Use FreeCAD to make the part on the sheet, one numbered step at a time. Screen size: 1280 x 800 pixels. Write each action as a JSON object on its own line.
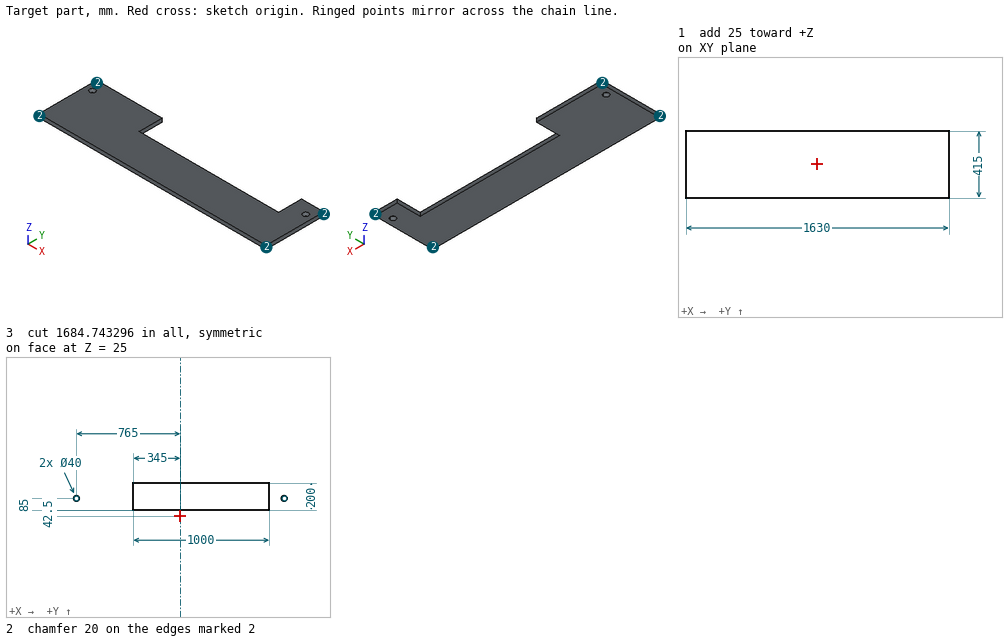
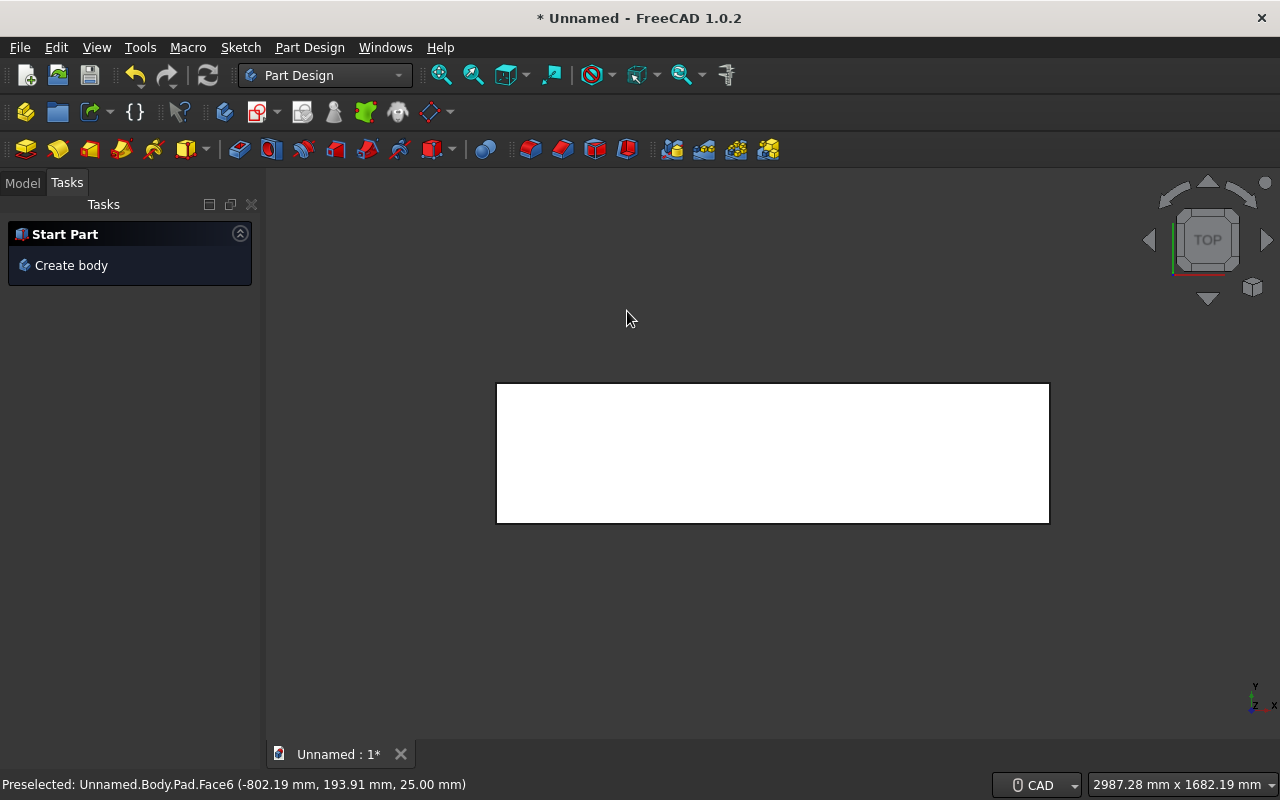
{"action": "scroll", "coordinate": [496, 382], "scroll_direction": "up", "scroll_amount": 8}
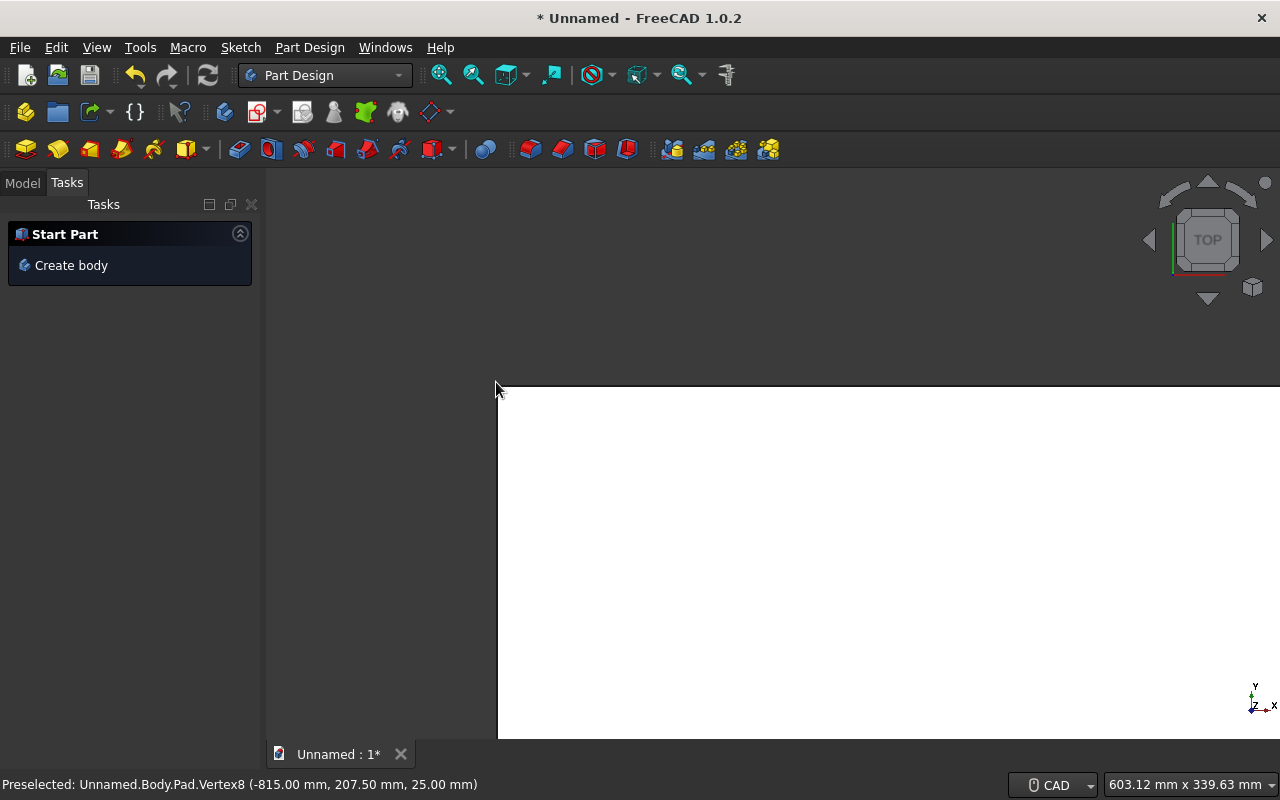
{"action": "left_click", "coordinate": [442, 76]}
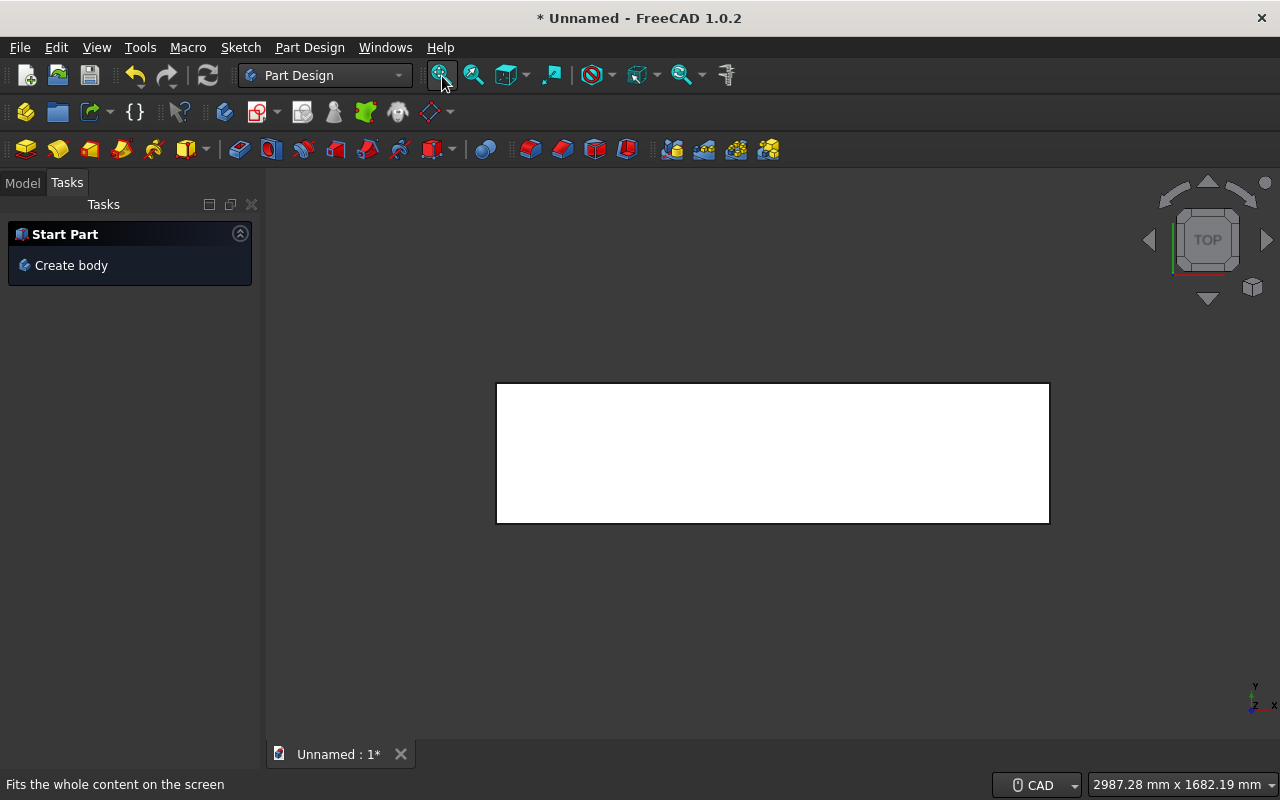
{"action": "key", "text": "1"}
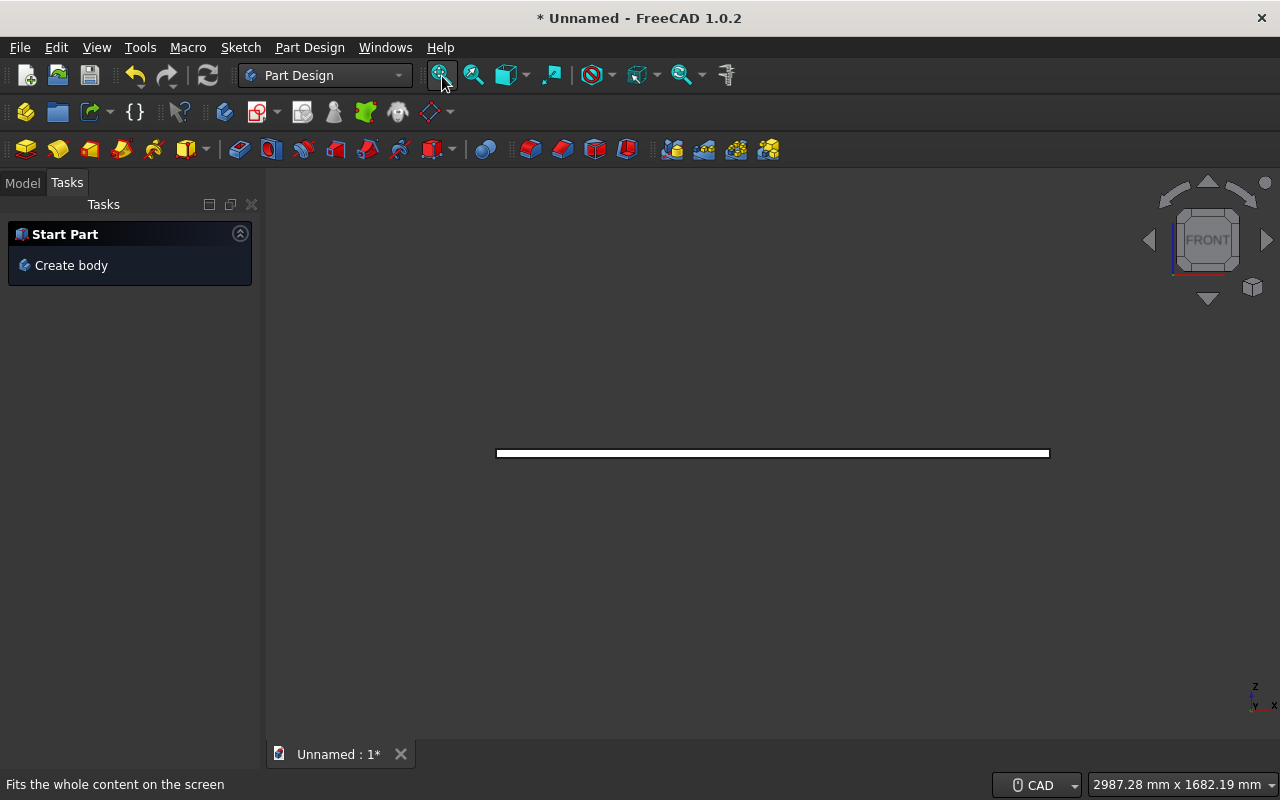
{"action": "scroll", "coordinate": [496, 453], "scroll_direction": "up", "scroll_amount": 8}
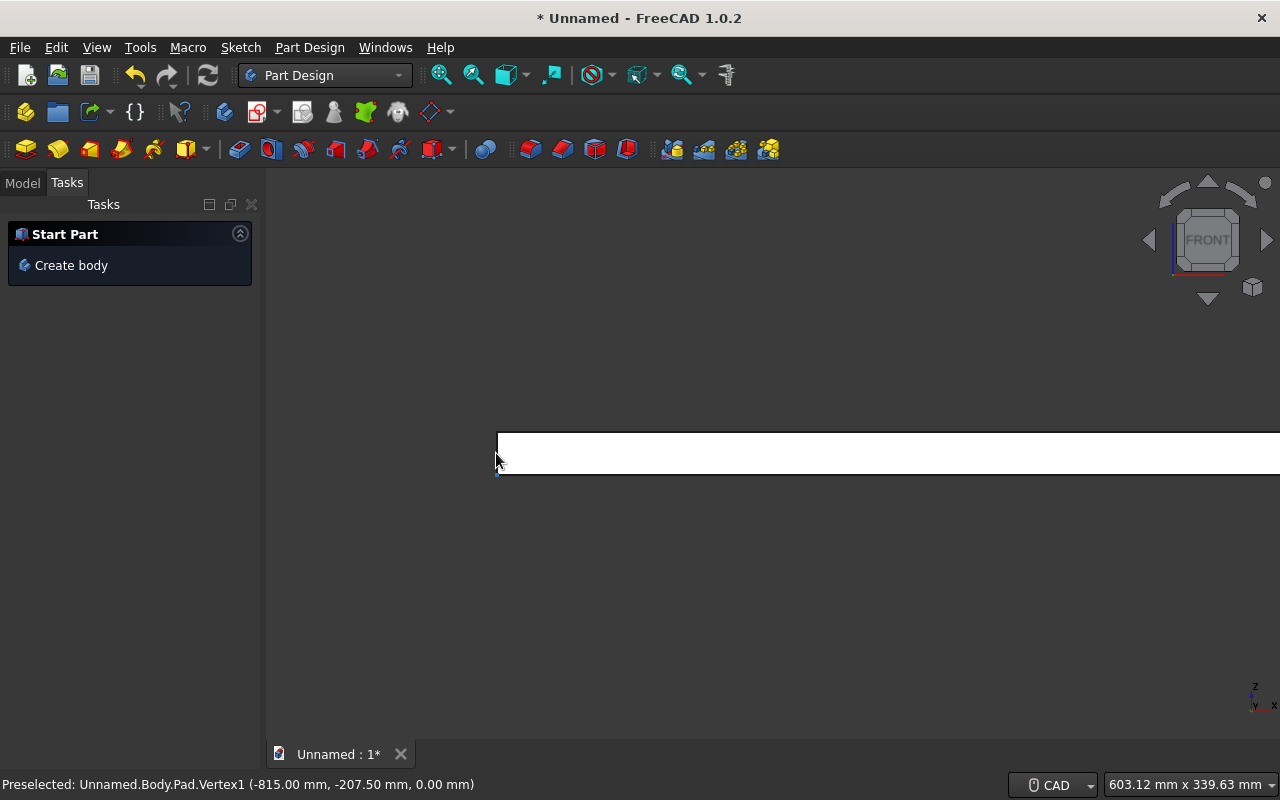
{"action": "left_click", "coordinate": [497, 453]}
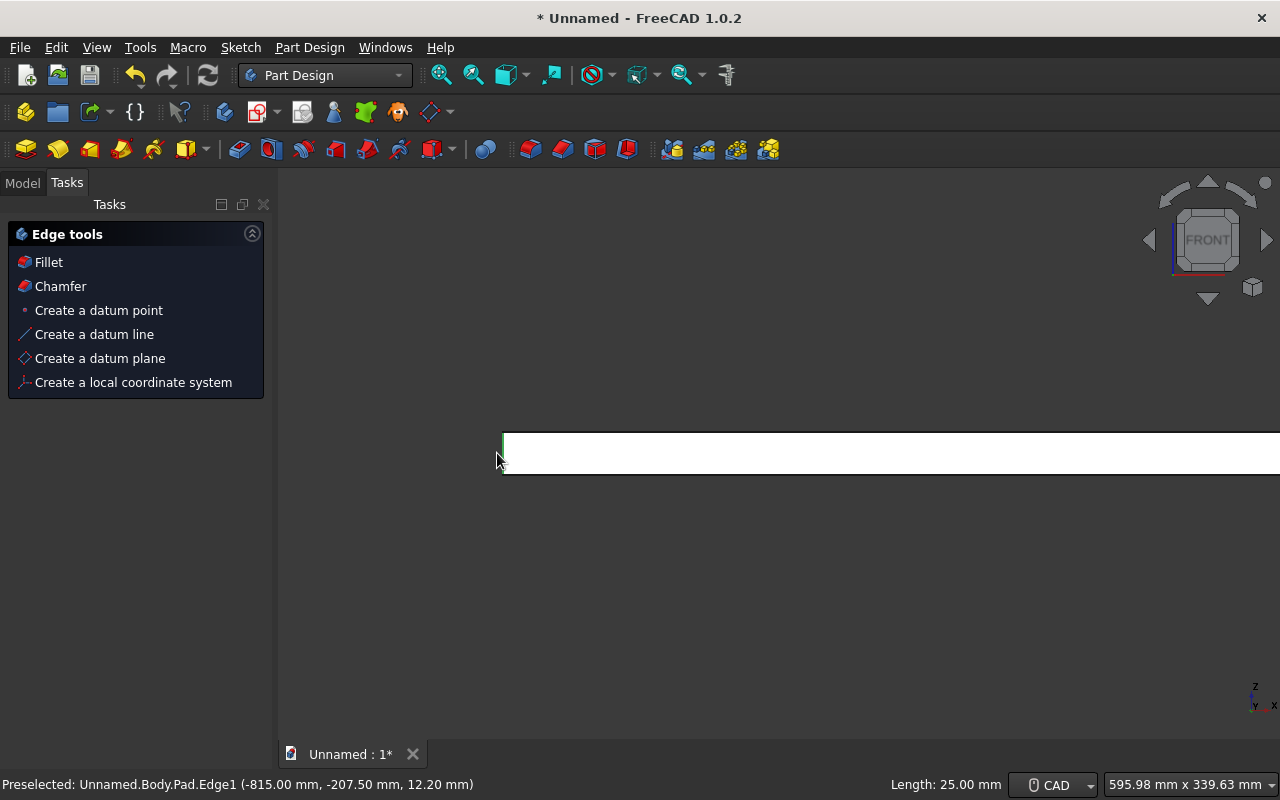
{"action": "left_click", "coordinate": [442, 76]}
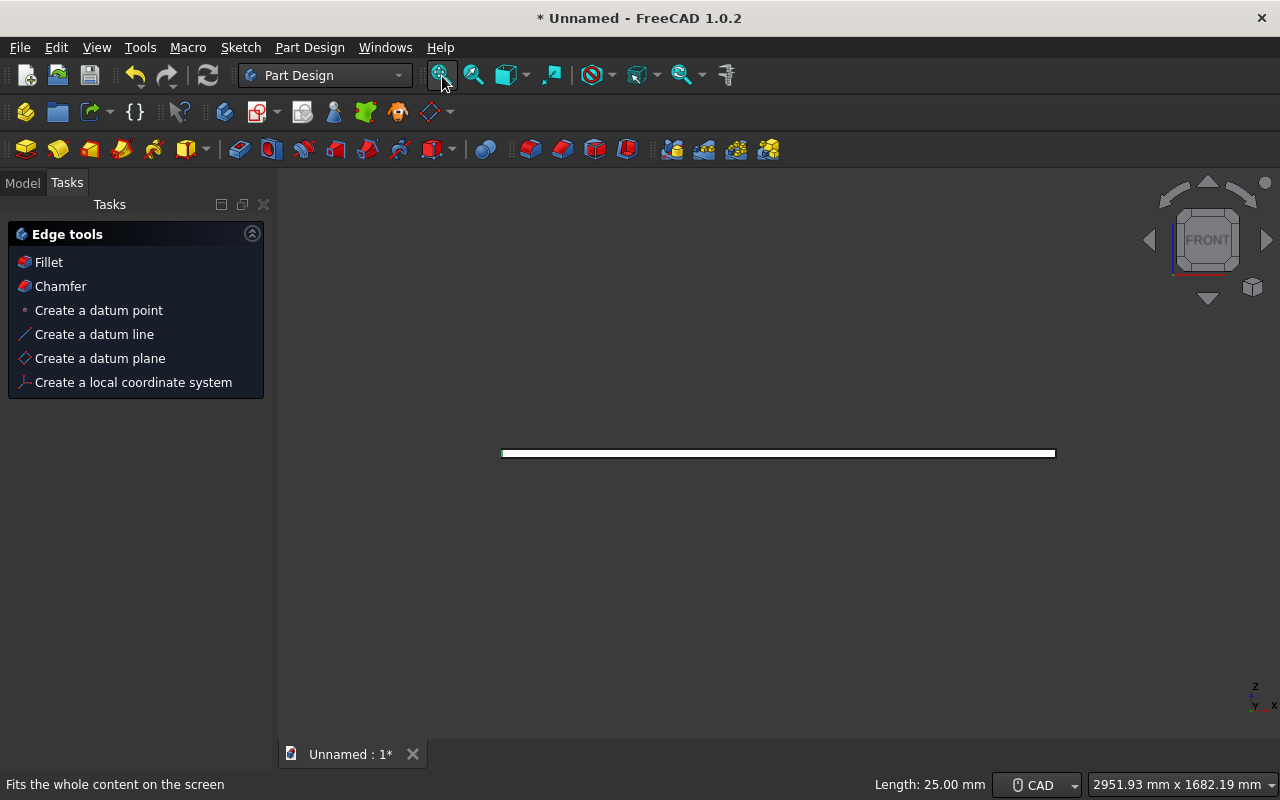
{"action": "key", "text": "3"}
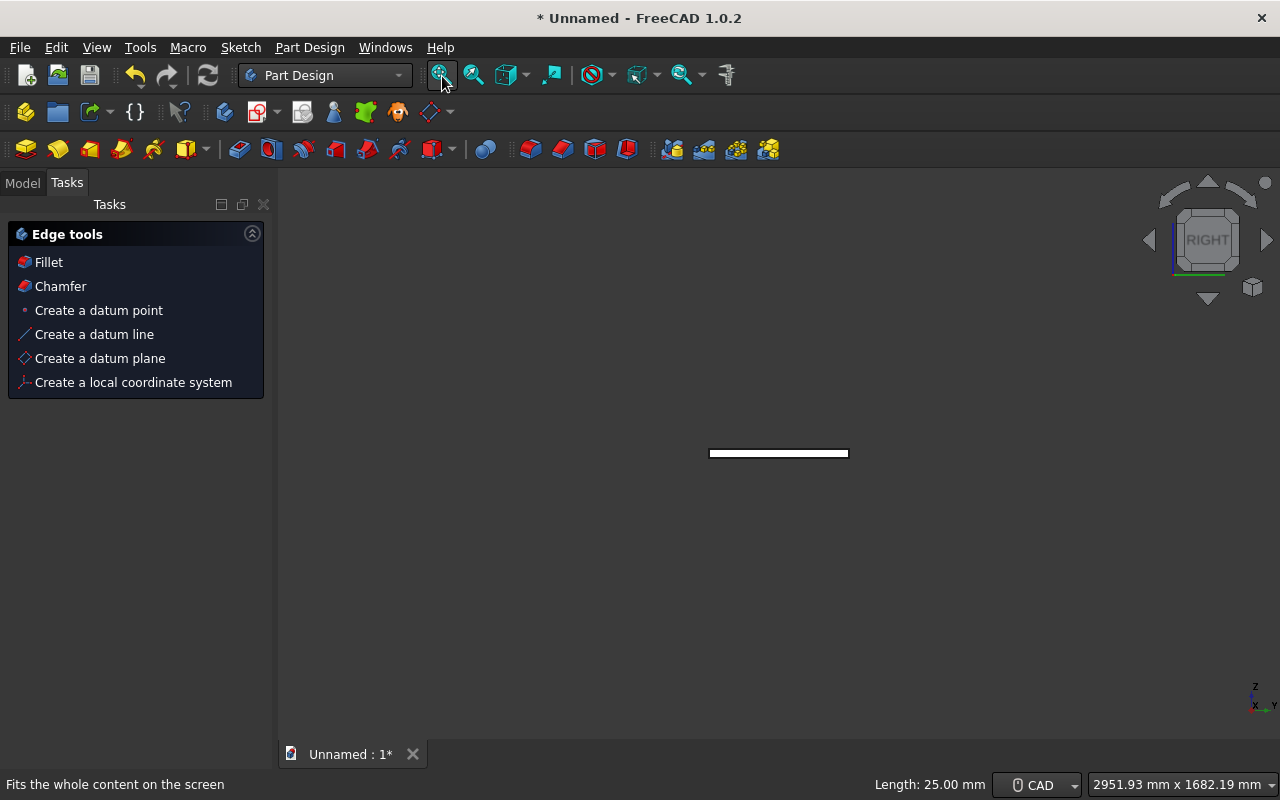
{"action": "left_click", "coordinate": [442, 76]}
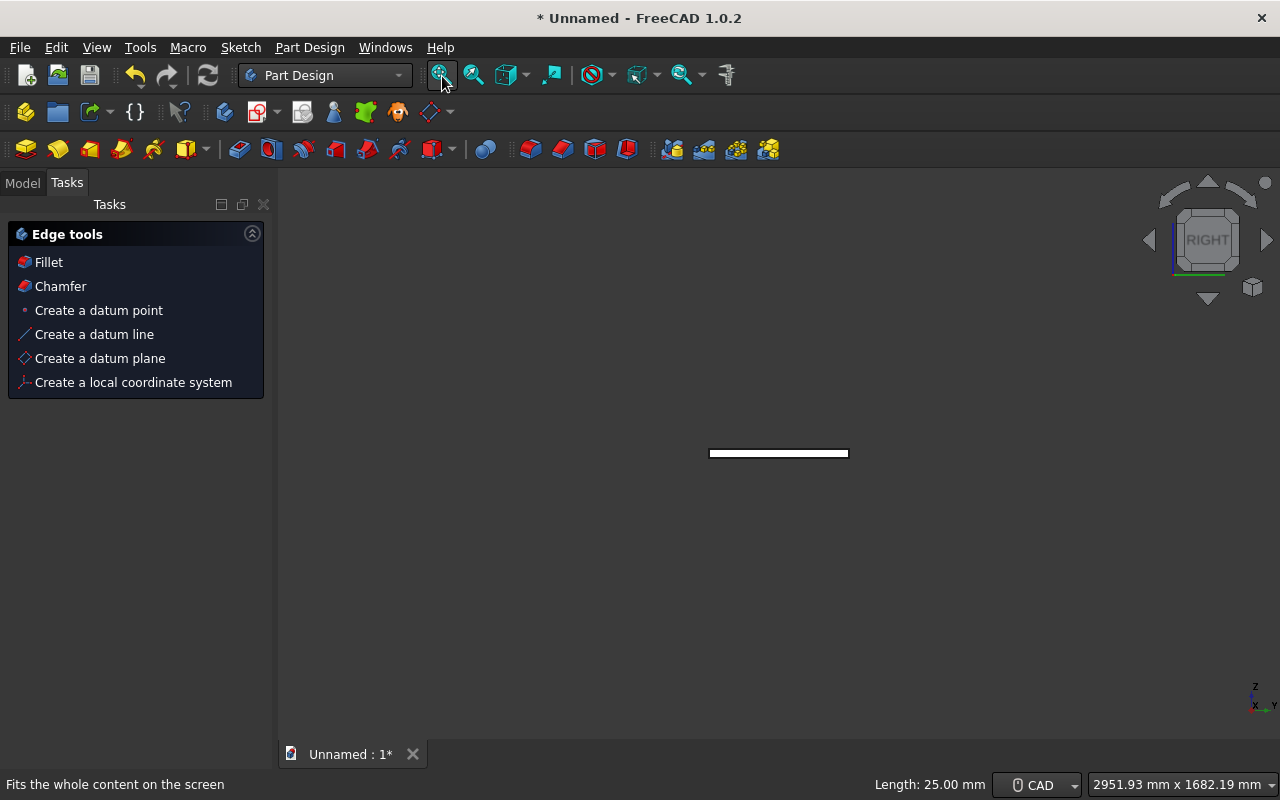
{"action": "scroll", "coordinate": [849, 452], "scroll_direction": "up", "scroll_amount": 8}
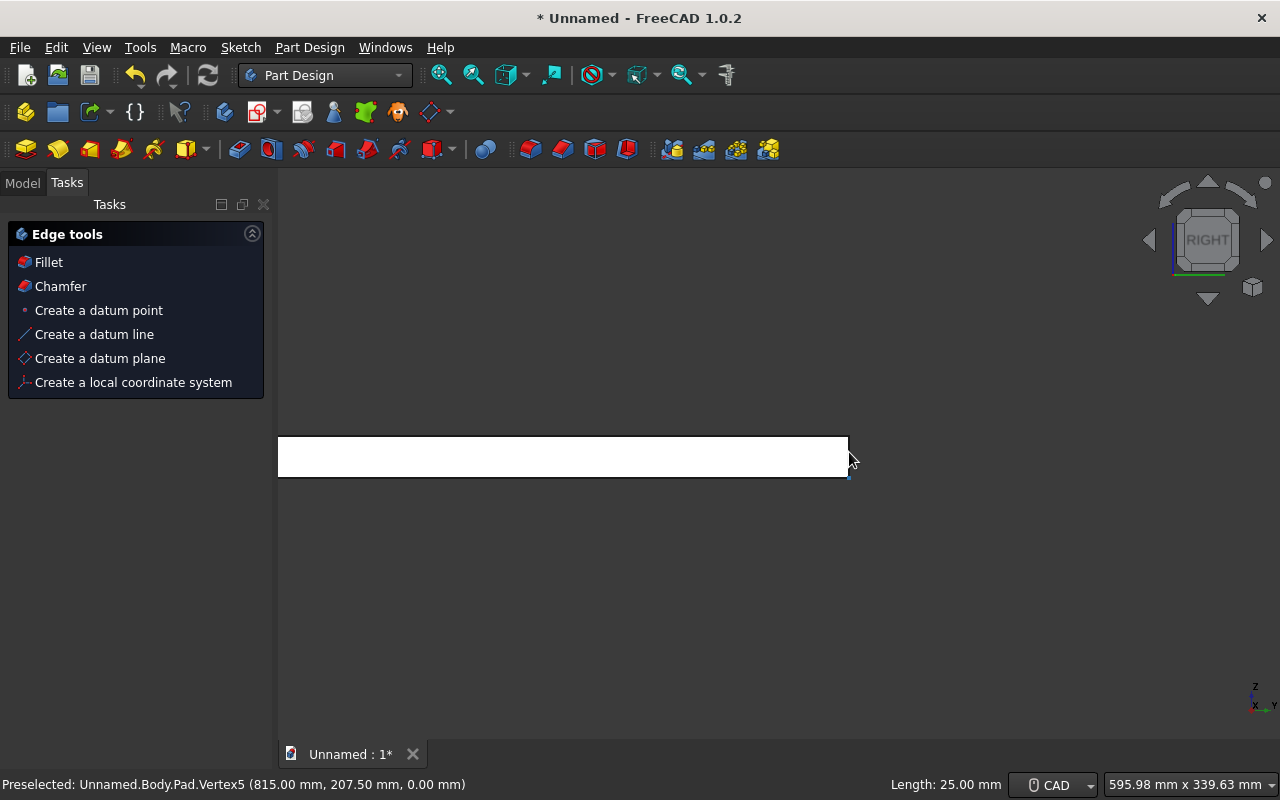
{"action": "left_click", "coordinate": [849, 456], "text": "ctrl"}